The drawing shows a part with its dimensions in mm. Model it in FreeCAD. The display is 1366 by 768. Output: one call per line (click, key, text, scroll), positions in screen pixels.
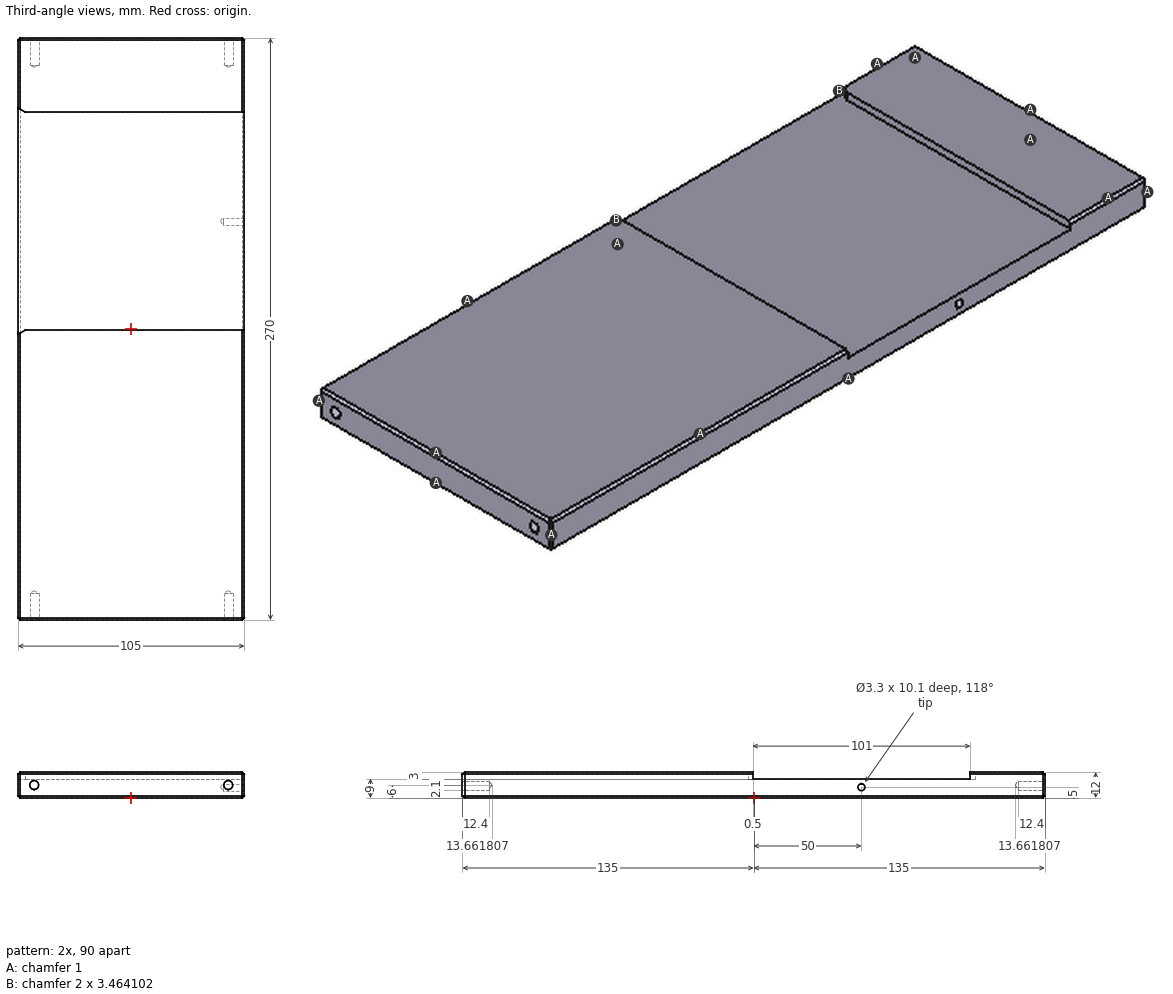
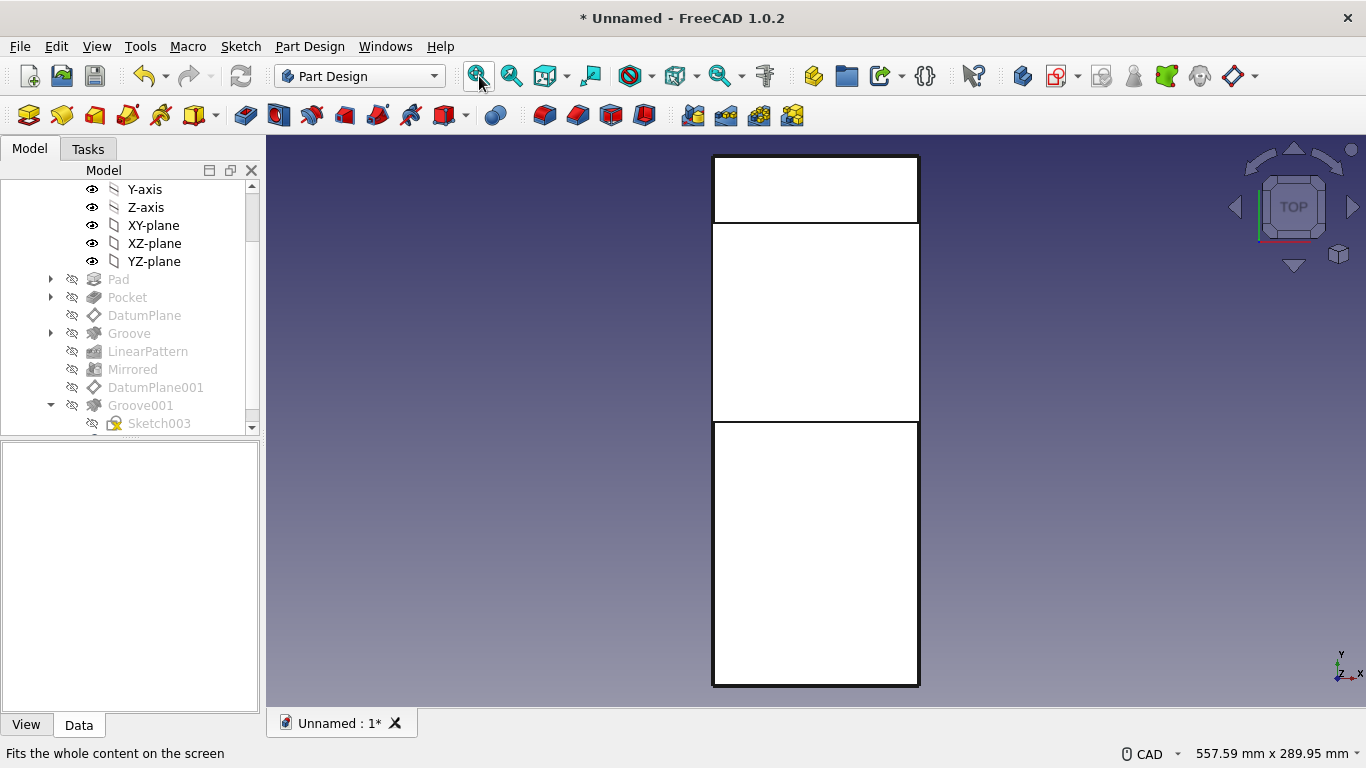
key(1)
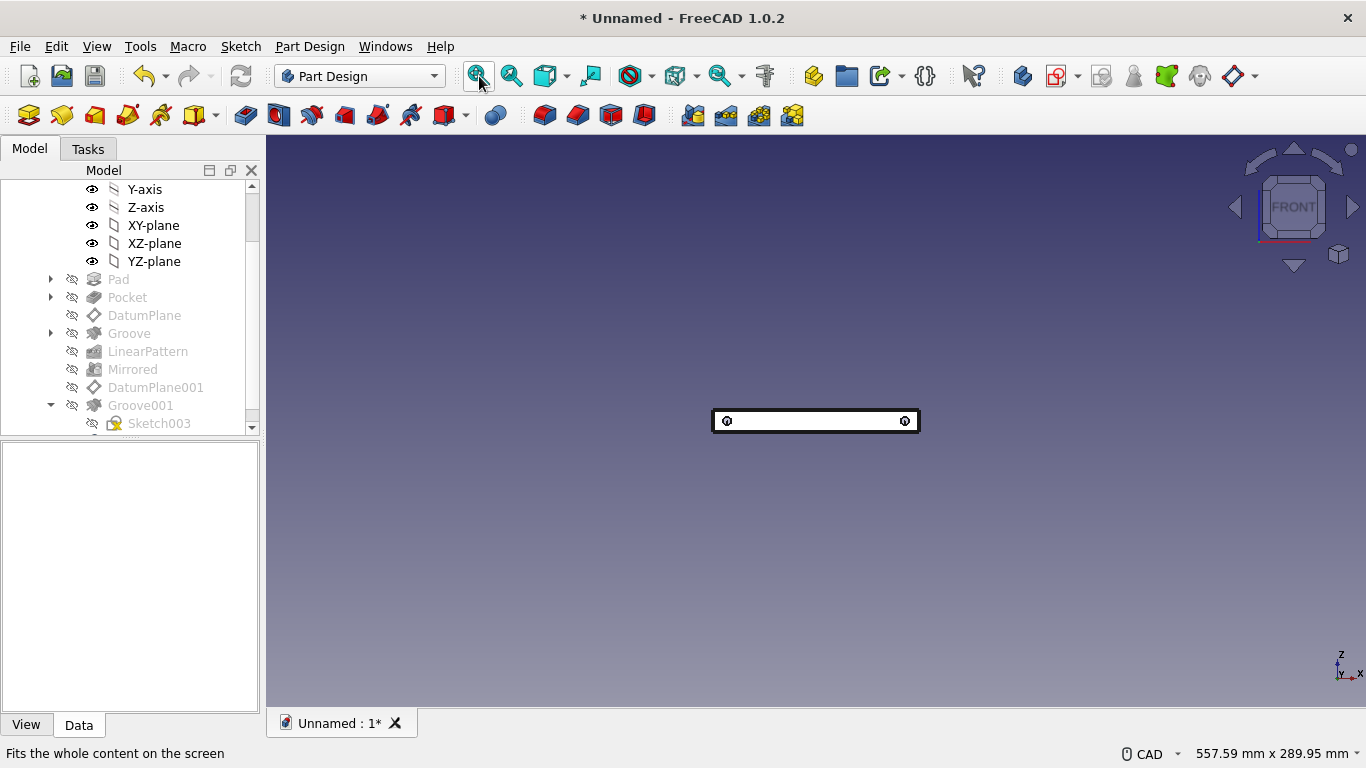
click(479, 76)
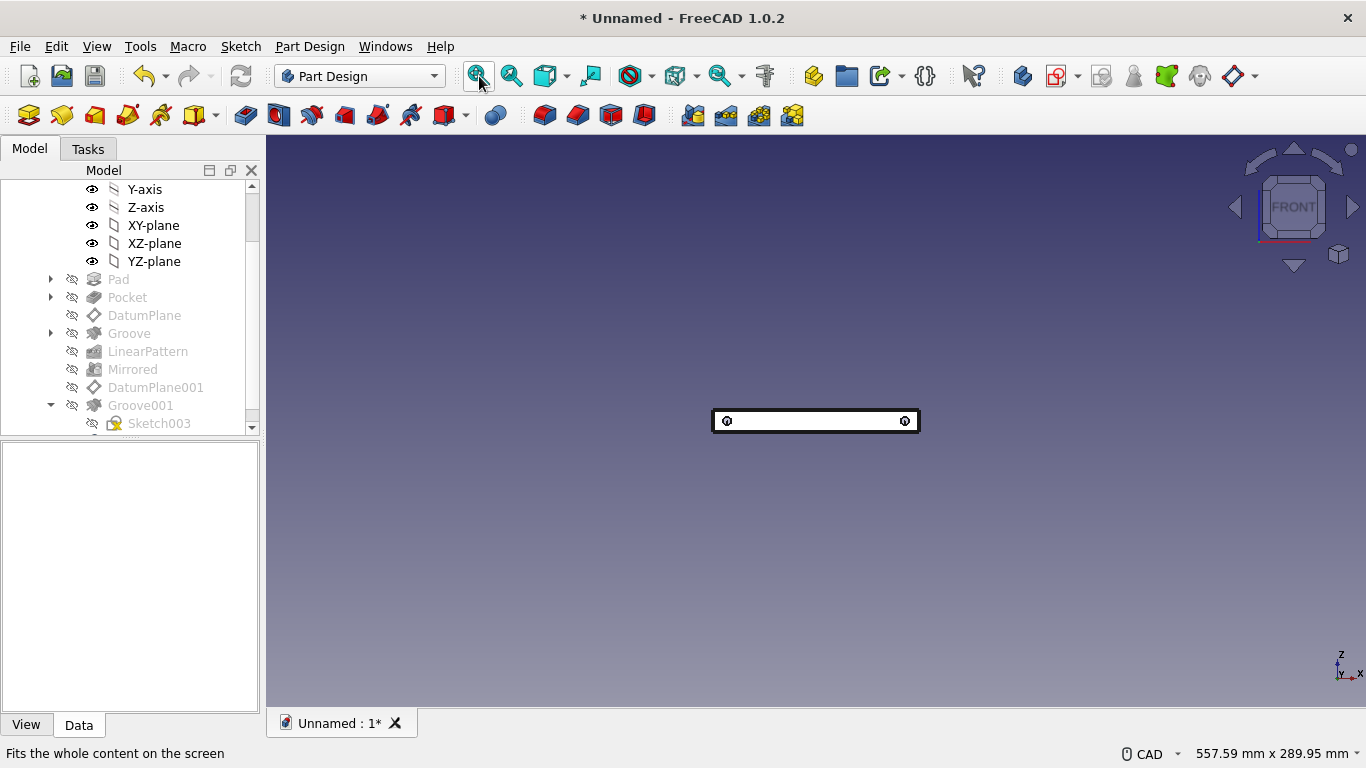
scroll(712, 412, up, 12)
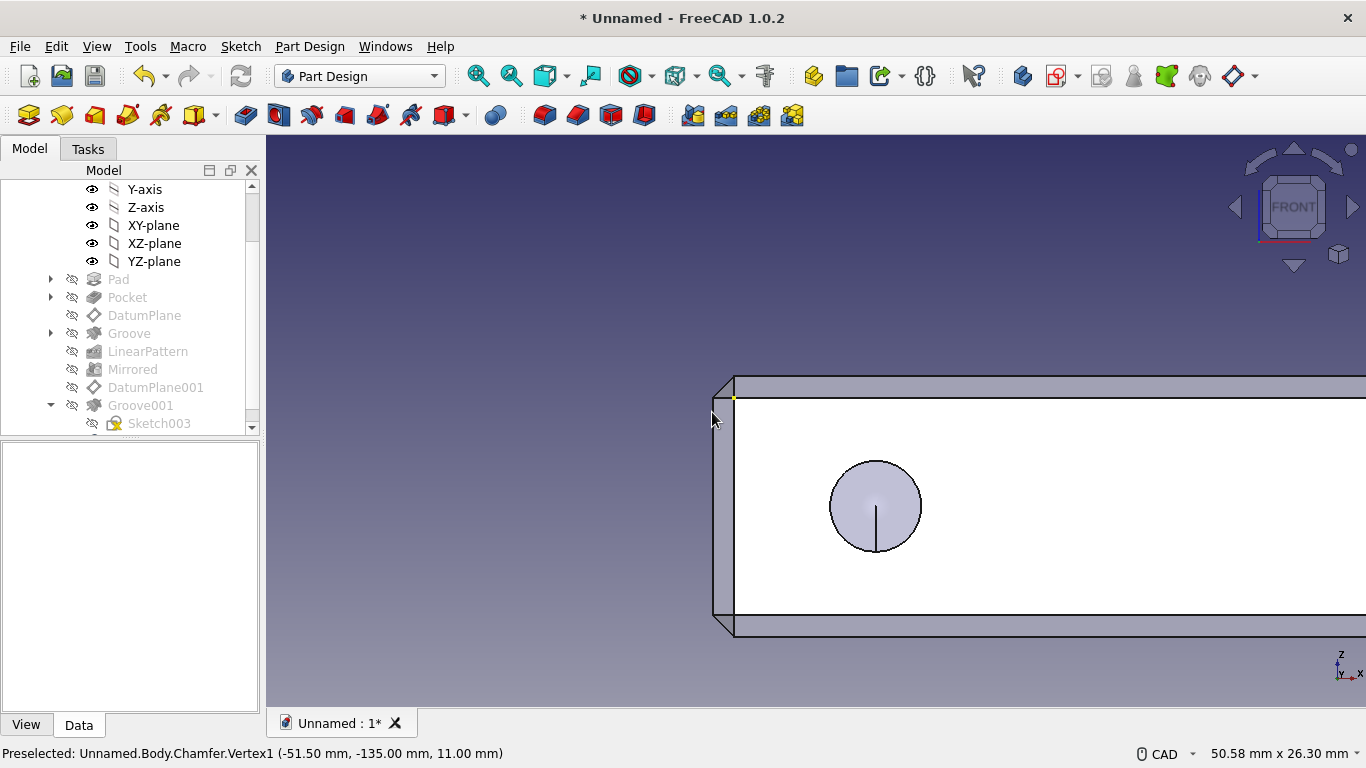
click(479, 76)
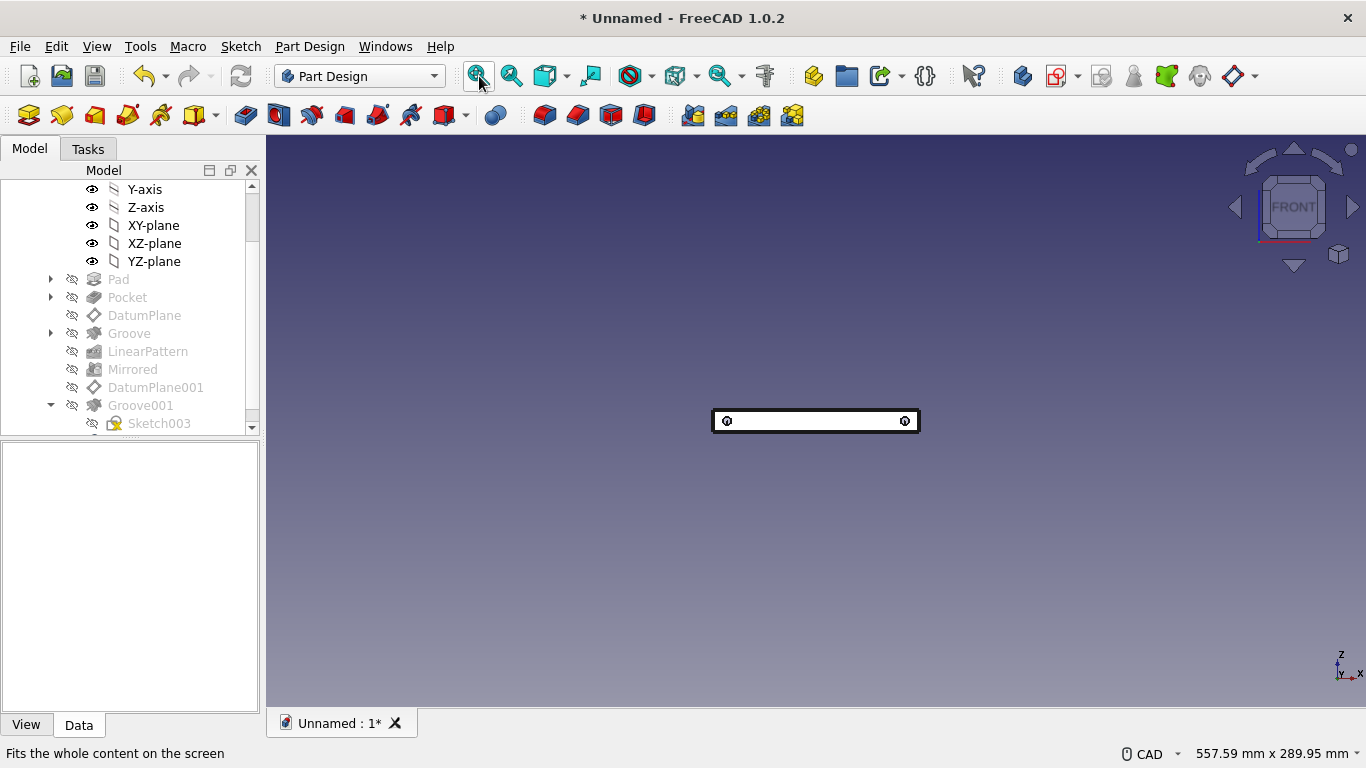
key(3)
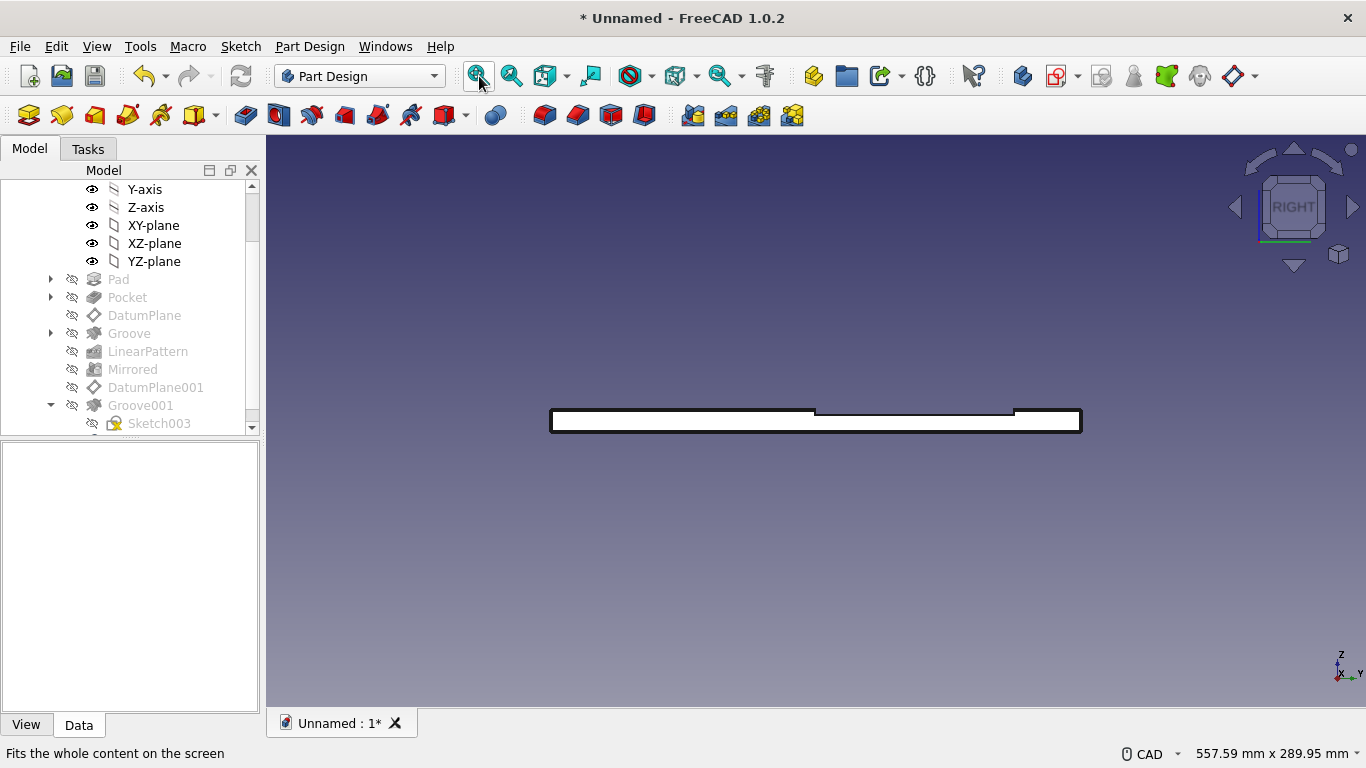
scroll(815, 412, up, 12)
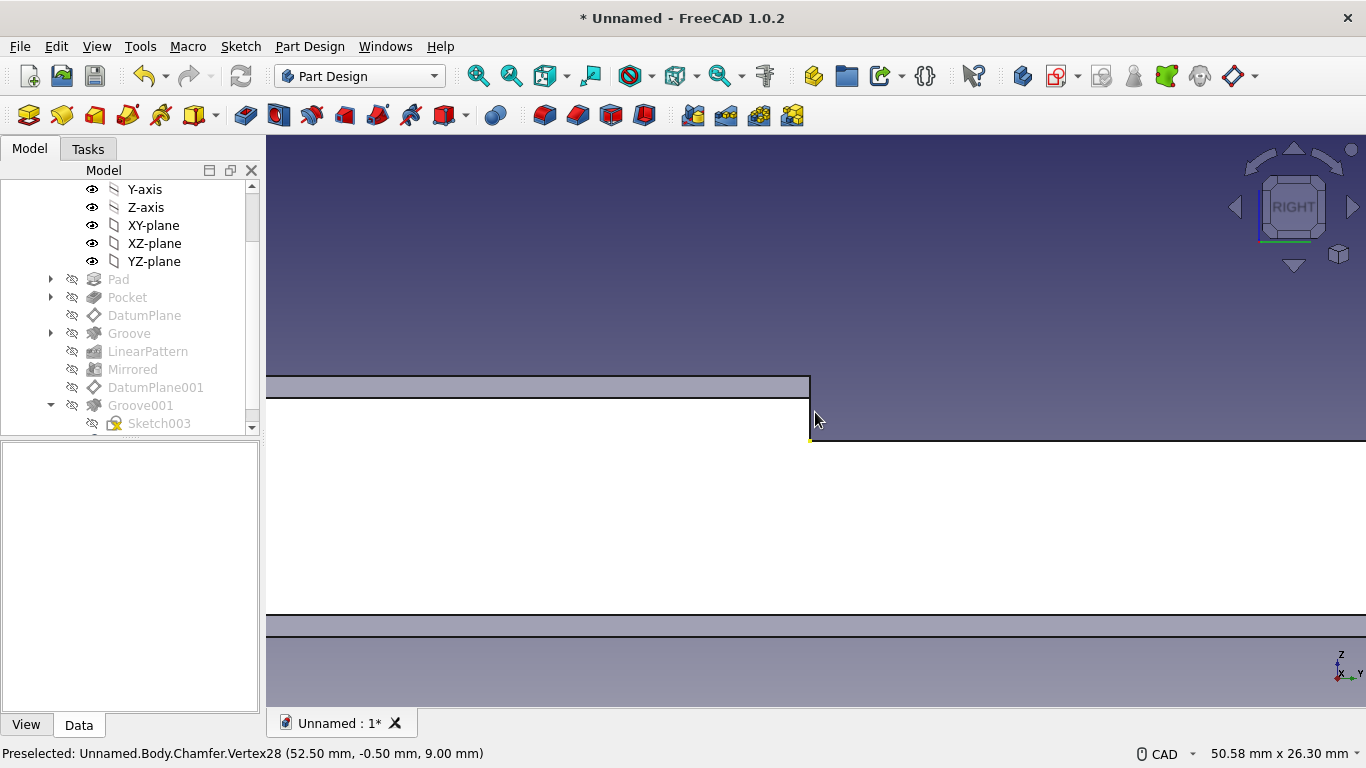
click(479, 76)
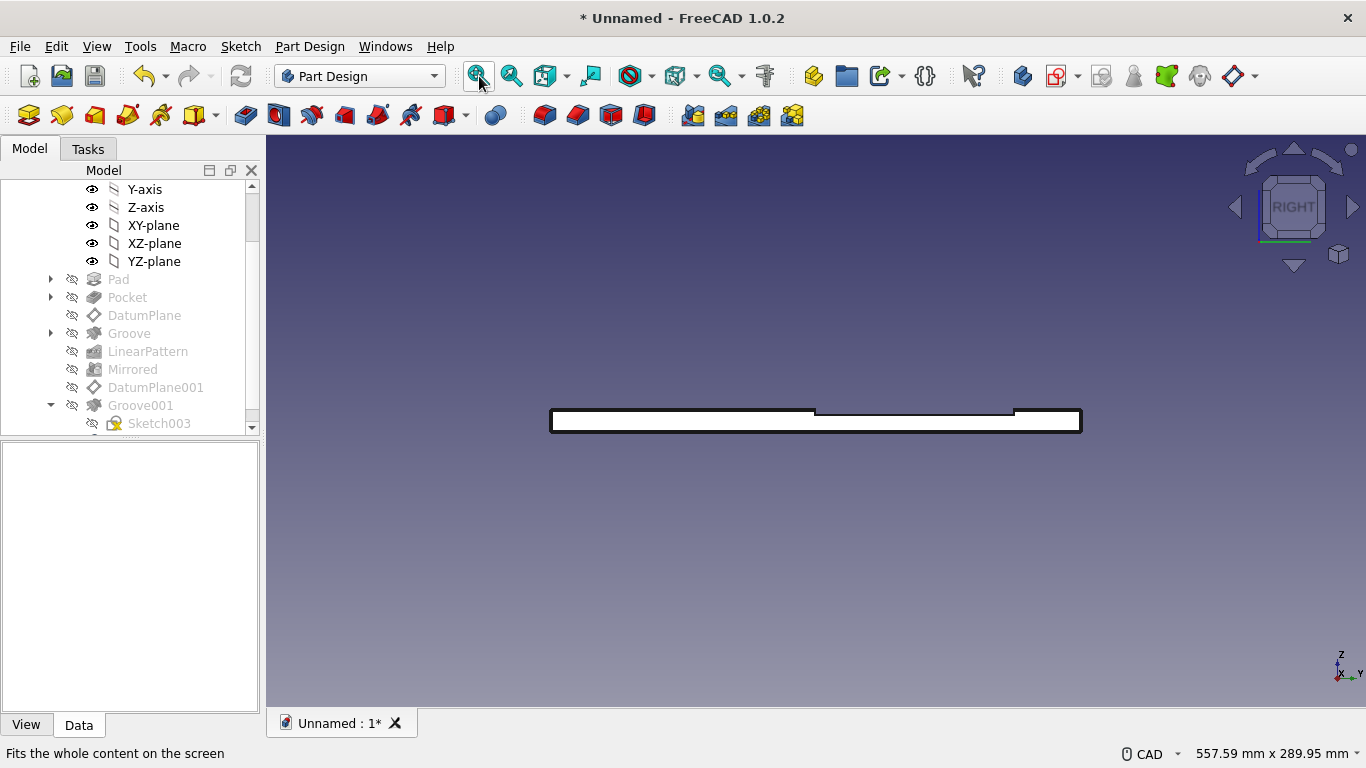
key(5)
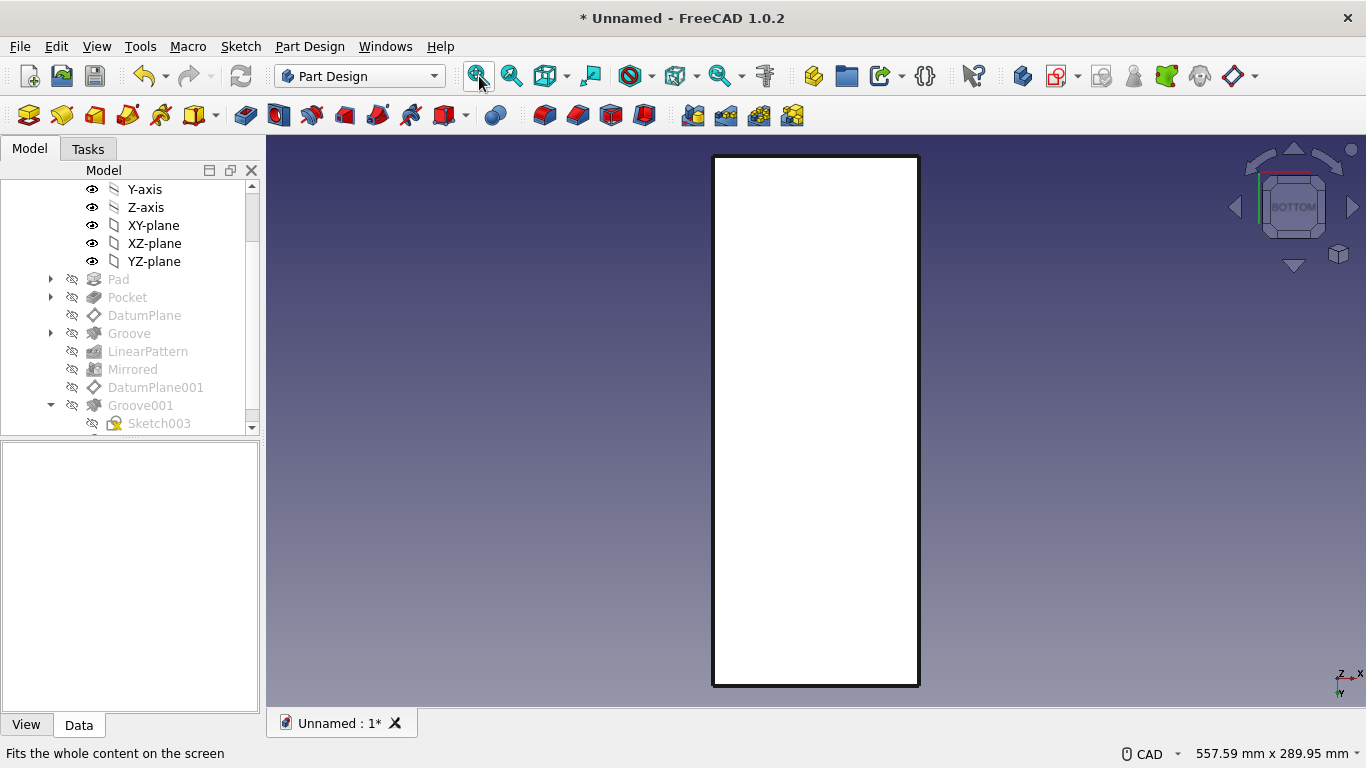
scroll(712, 419, up, 12)